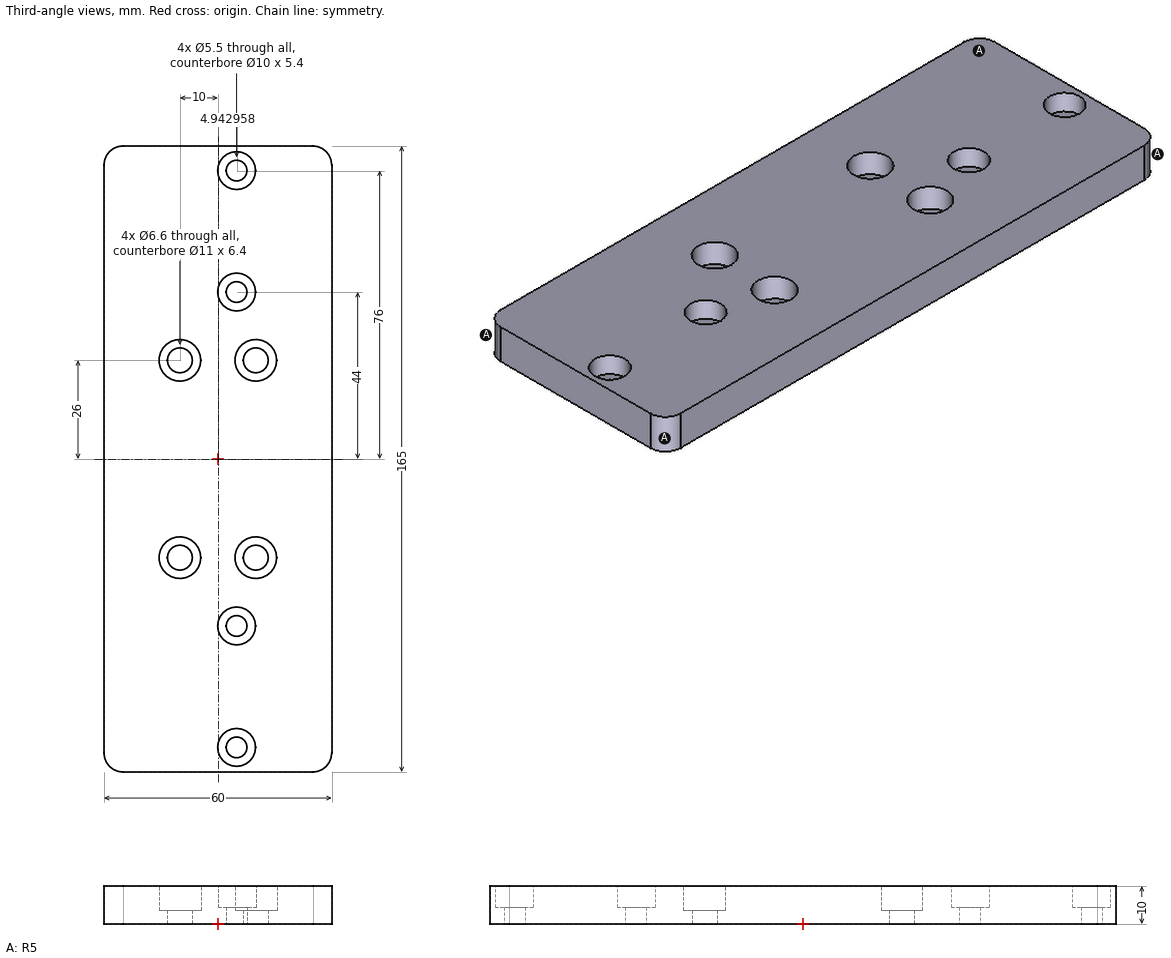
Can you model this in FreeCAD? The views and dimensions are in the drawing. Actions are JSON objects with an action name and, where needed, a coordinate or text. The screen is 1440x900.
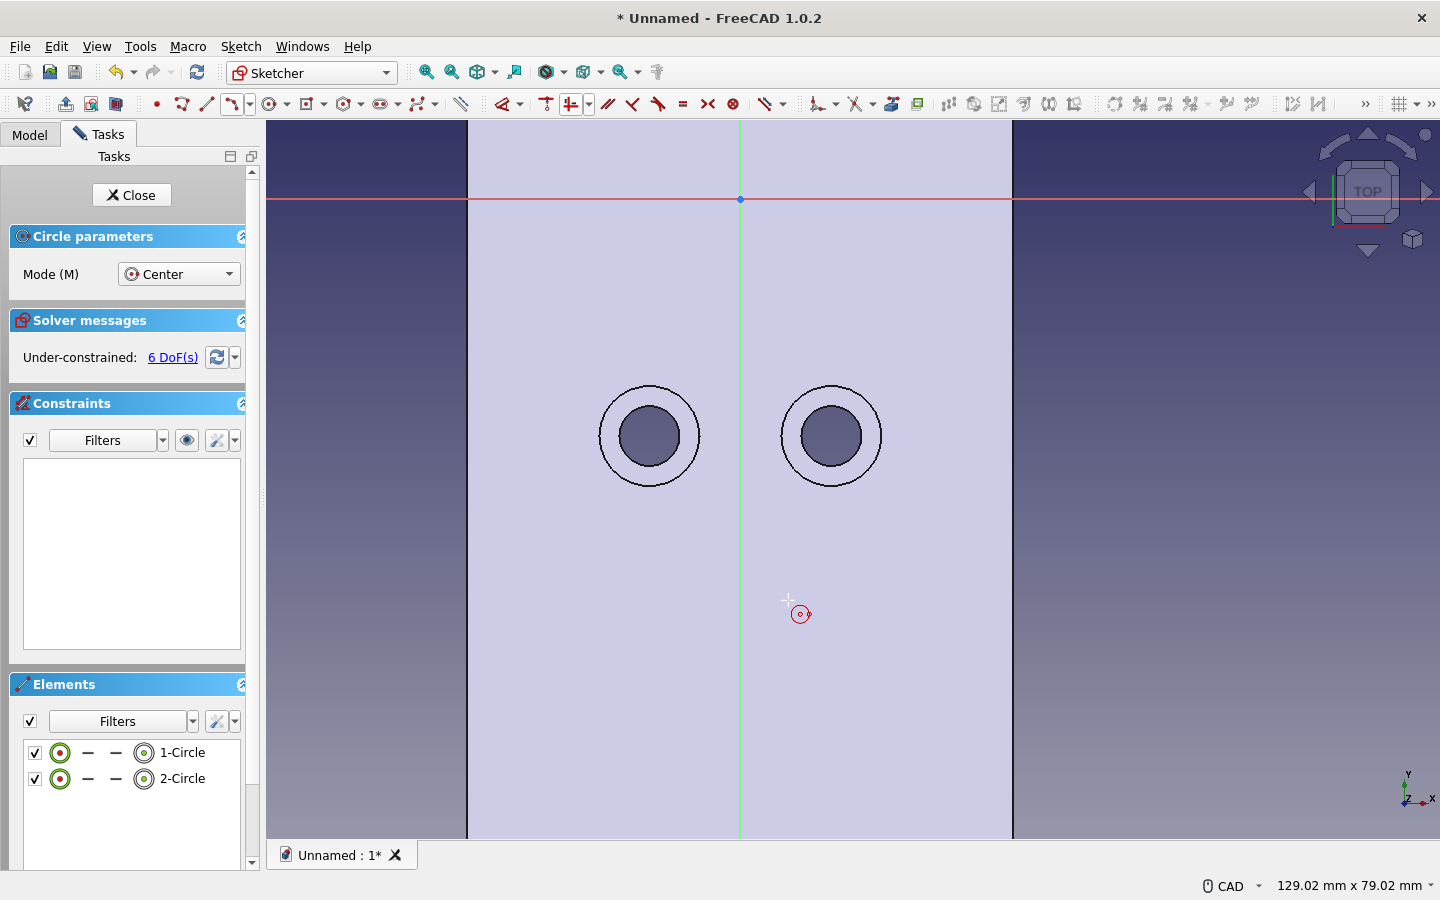
{"action": "left_click", "coordinate": [785, 600]}
{"action": "left_click", "coordinate": [803, 582]}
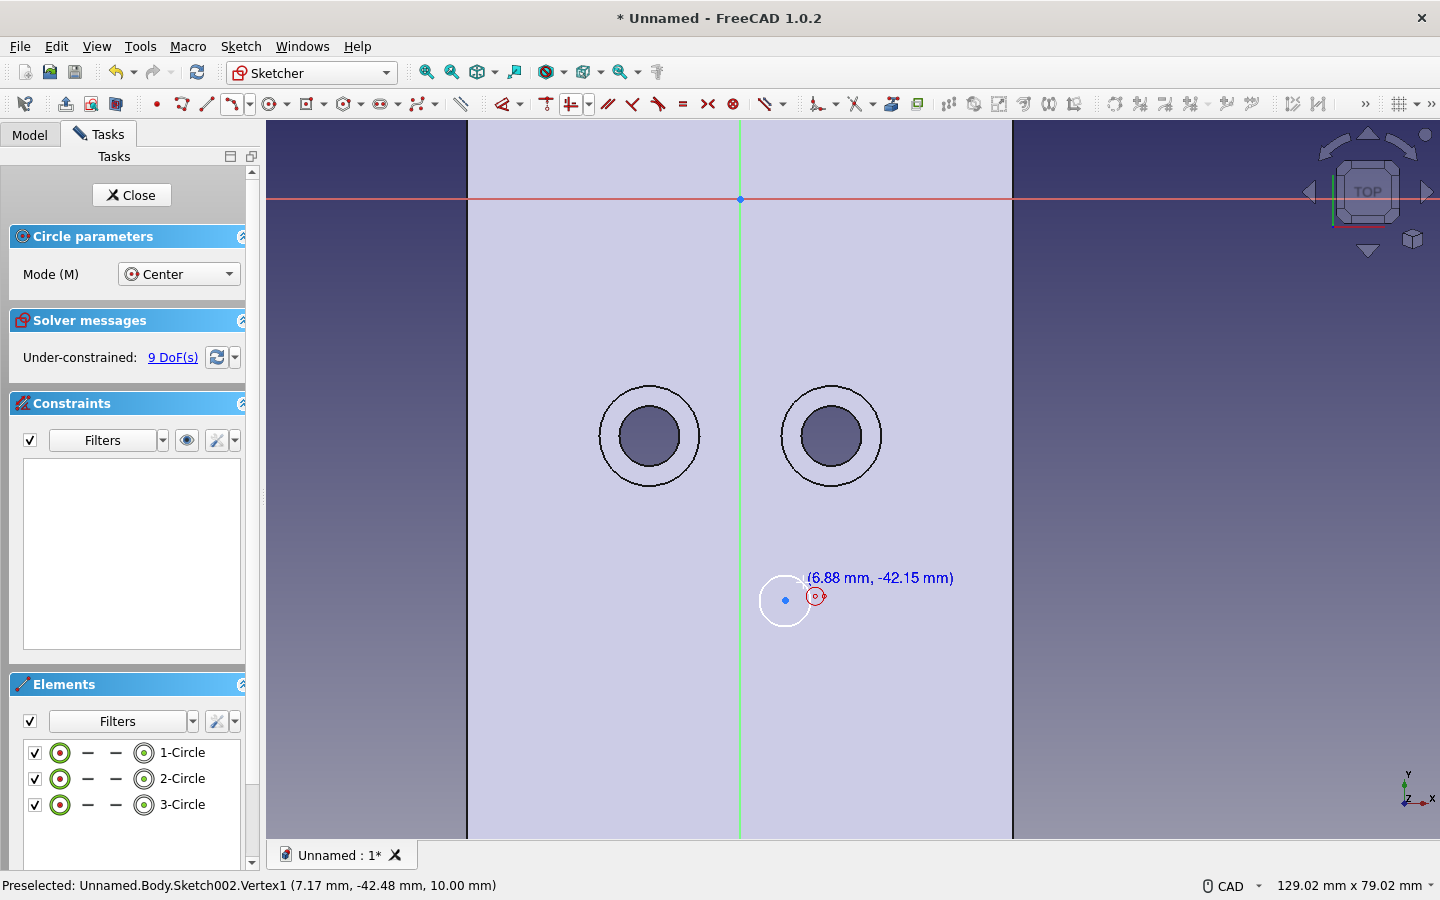
{"action": "scroll", "coordinate": [788, 600], "scroll_direction": "down", "scroll_amount": 6}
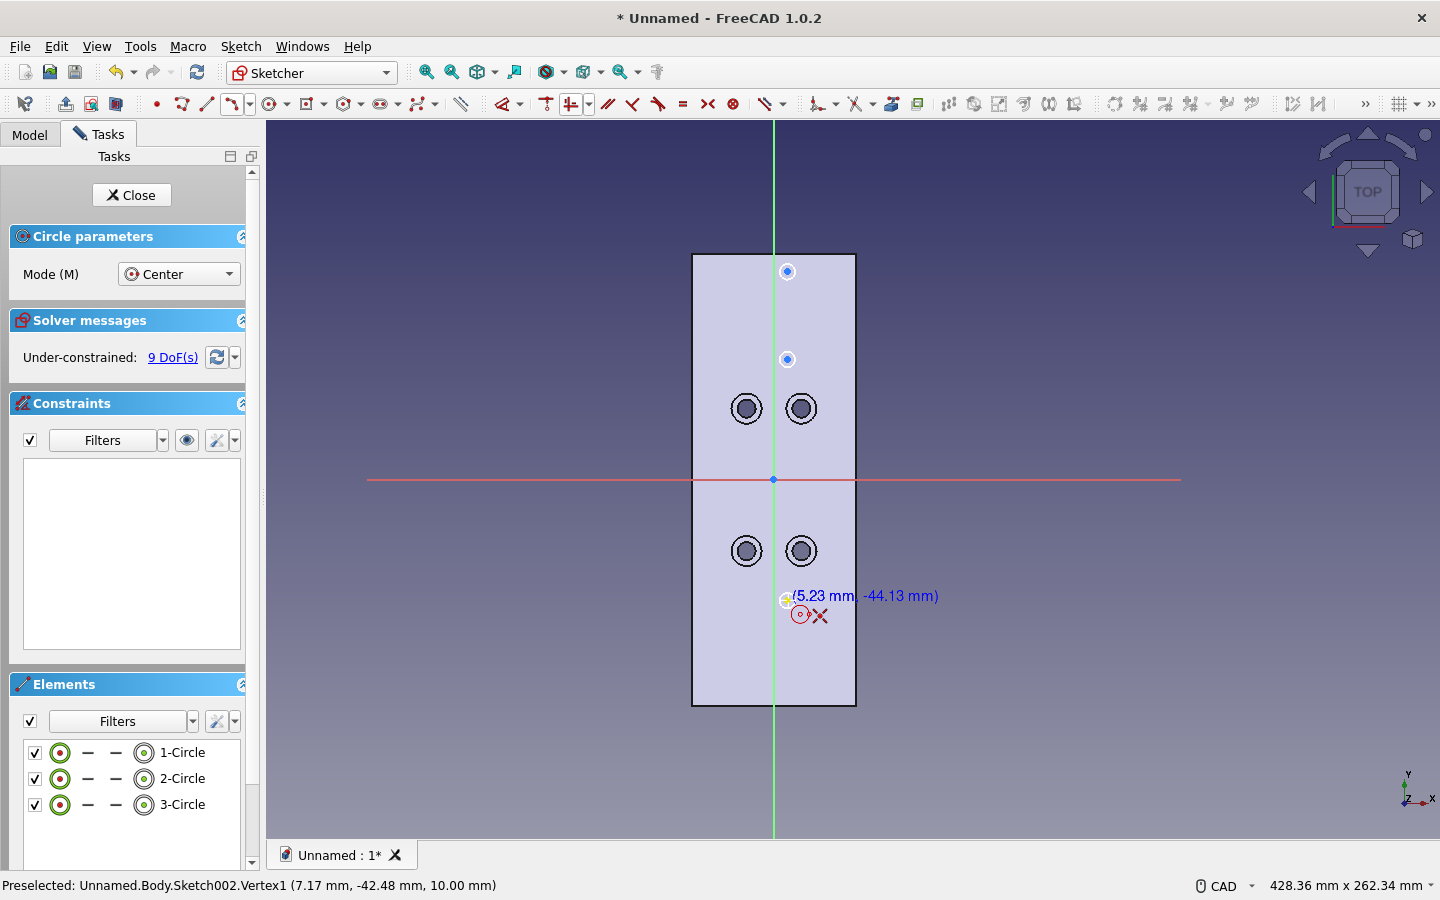
{"action": "scroll", "coordinate": [788, 688], "scroll_direction": "up", "scroll_amount": 6}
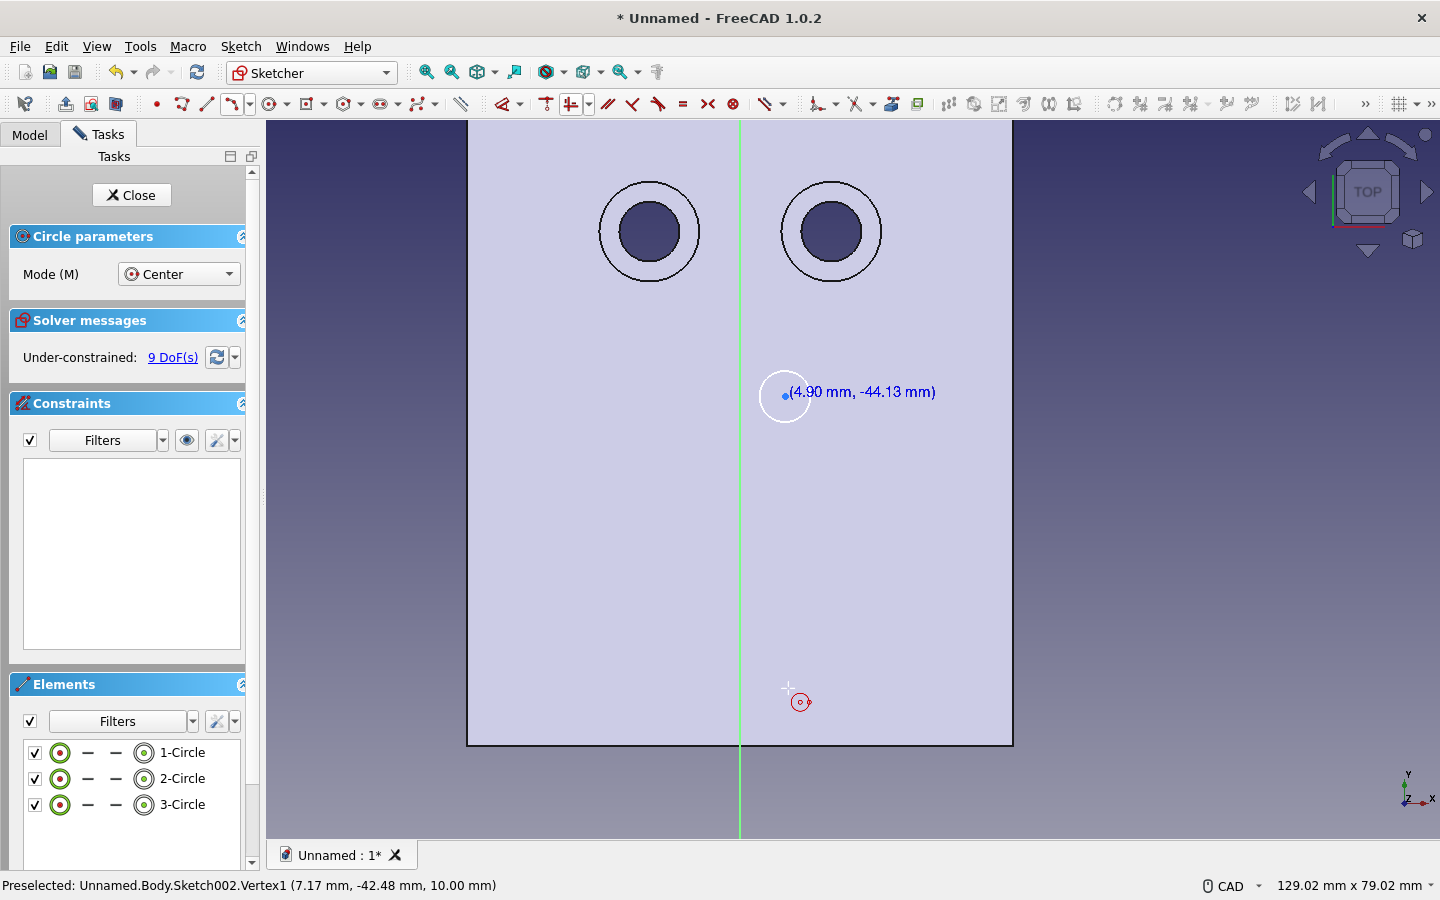
{"action": "left_click", "coordinate": [785, 687]}
{"action": "left_click", "coordinate": [803, 669]}
{"action": "key", "text": "Escape"}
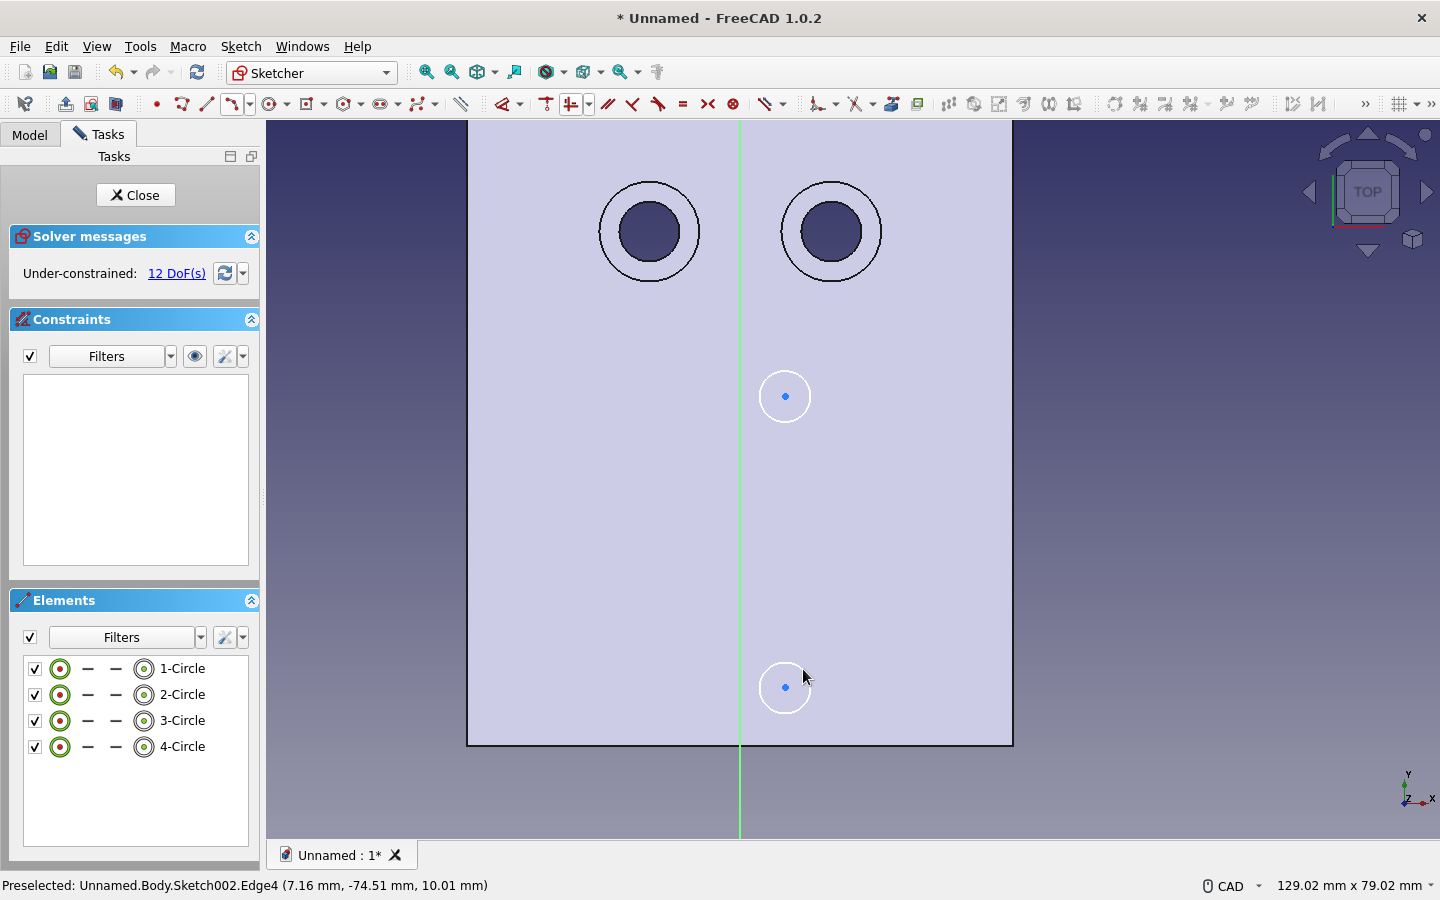
{"action": "scroll", "coordinate": [788, 688], "scroll_direction": "down", "scroll_amount": 6}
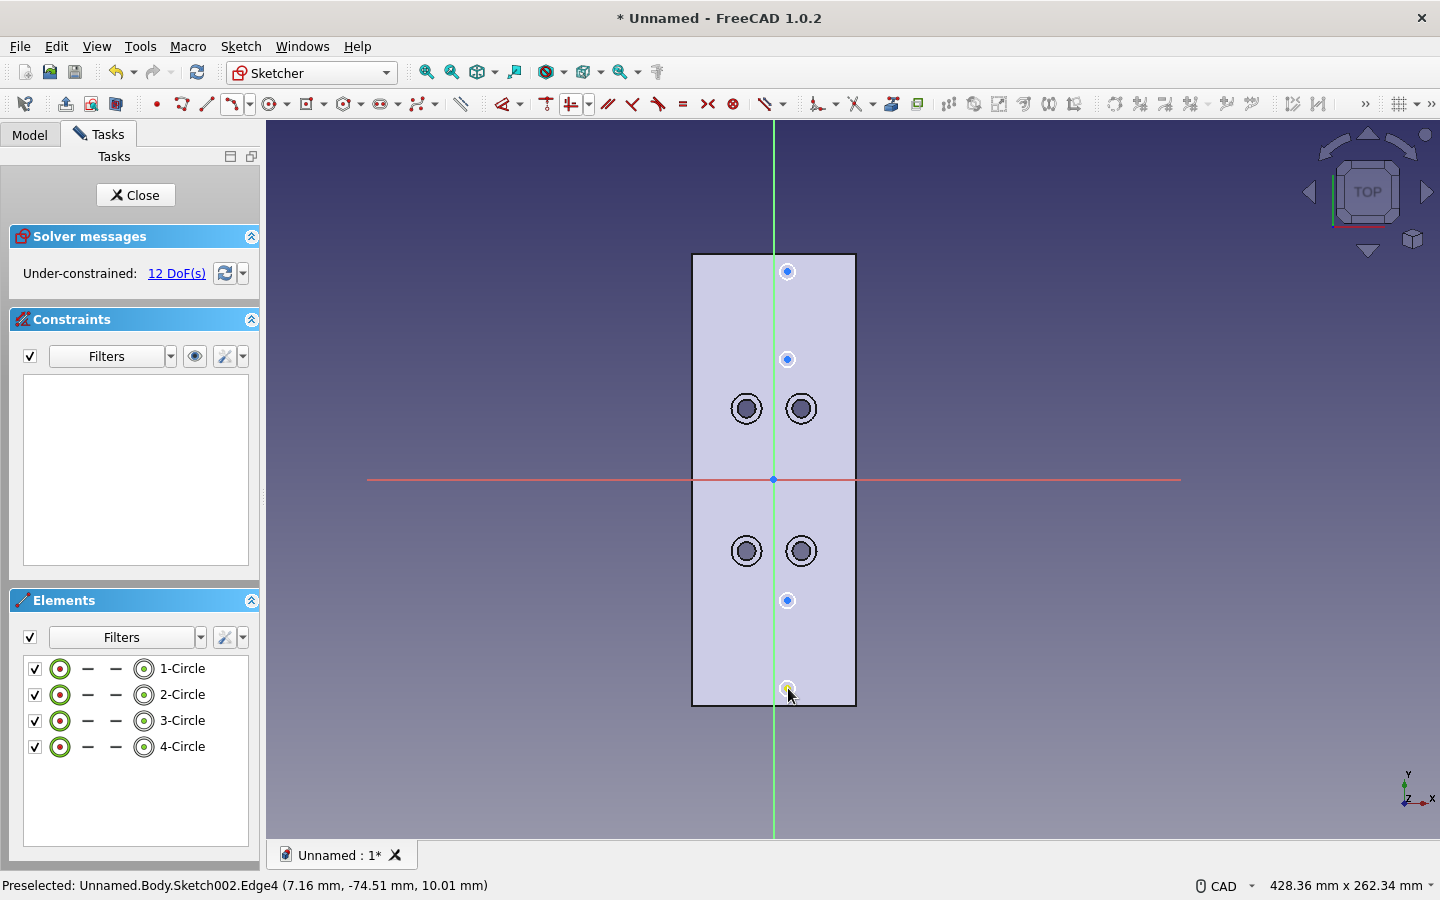
{"action": "scroll", "coordinate": [793, 266], "scroll_direction": "up", "scroll_amount": 3}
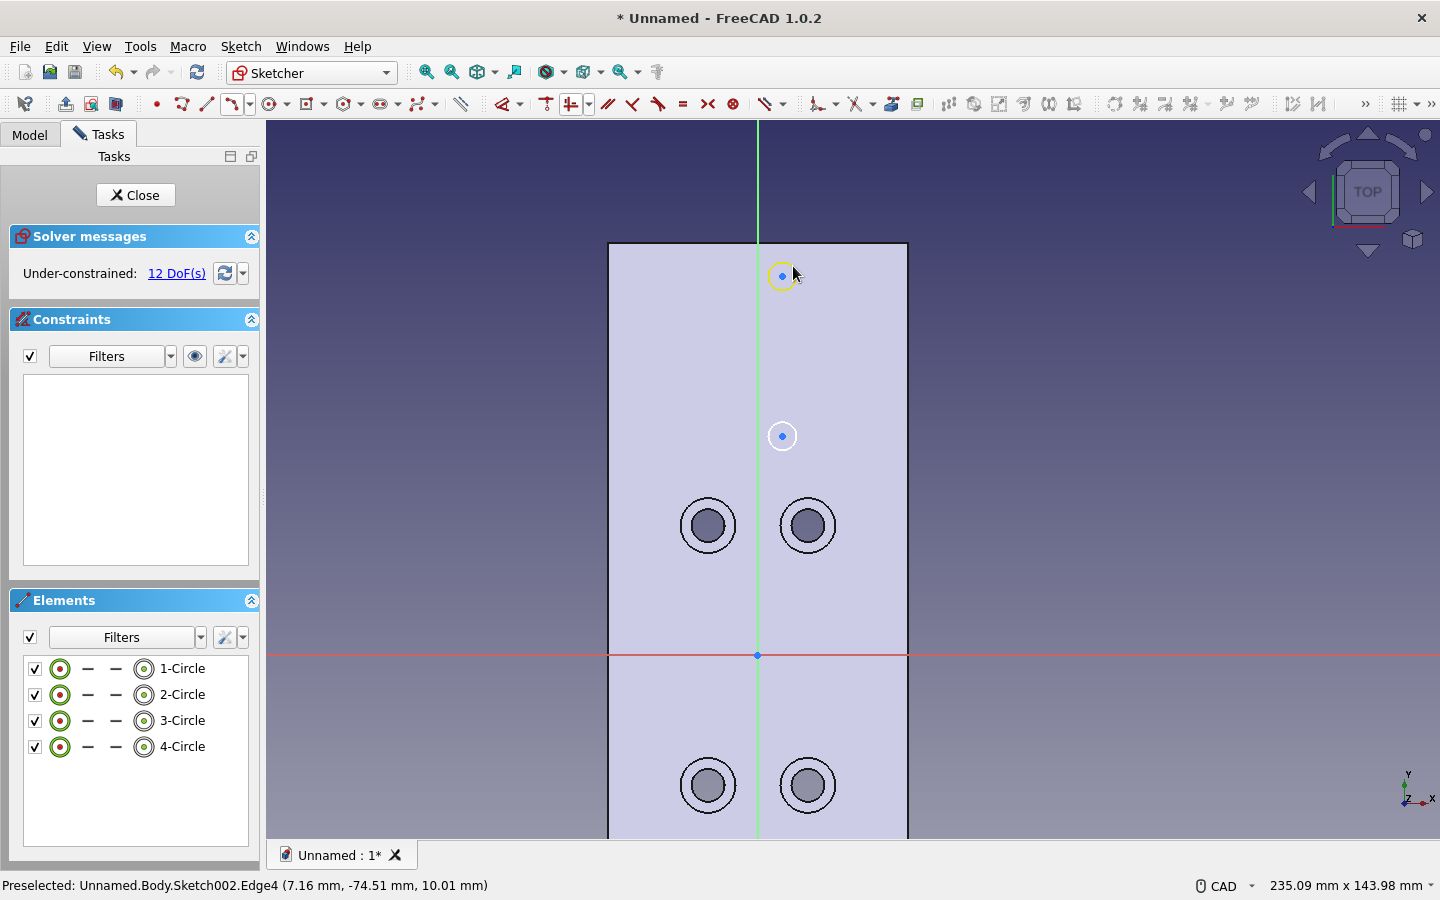
{"action": "left_click", "coordinate": [792, 267]}